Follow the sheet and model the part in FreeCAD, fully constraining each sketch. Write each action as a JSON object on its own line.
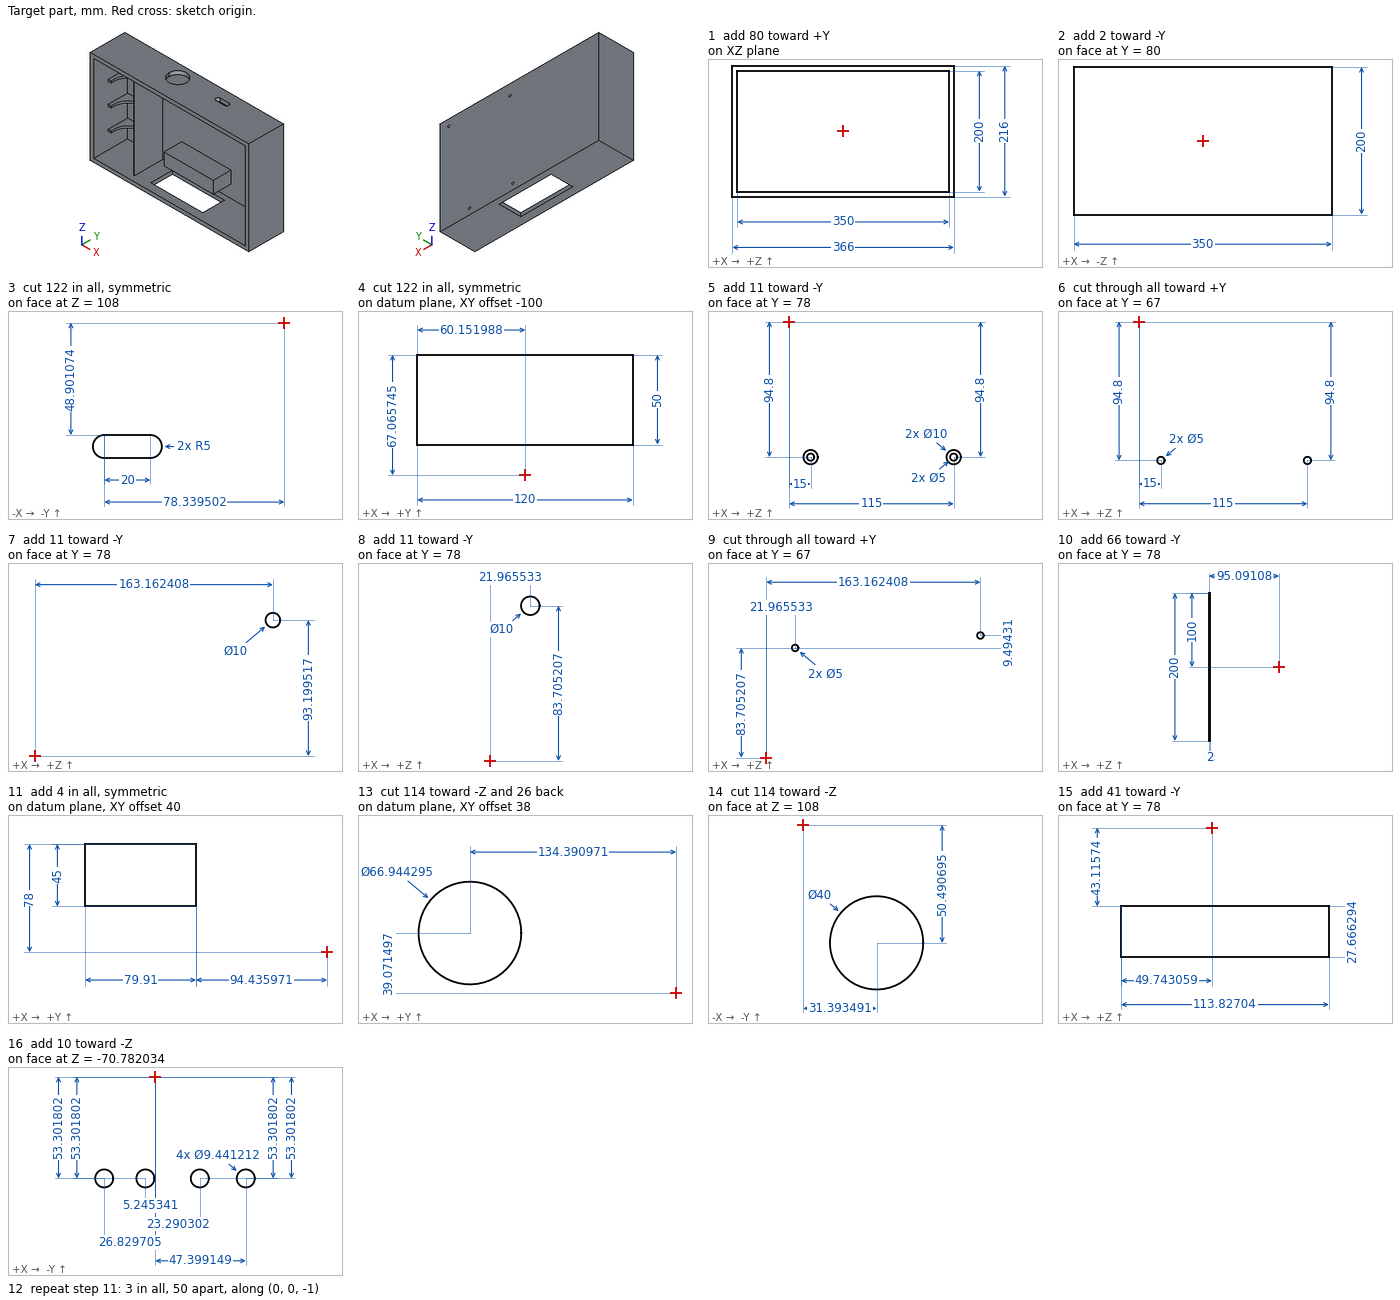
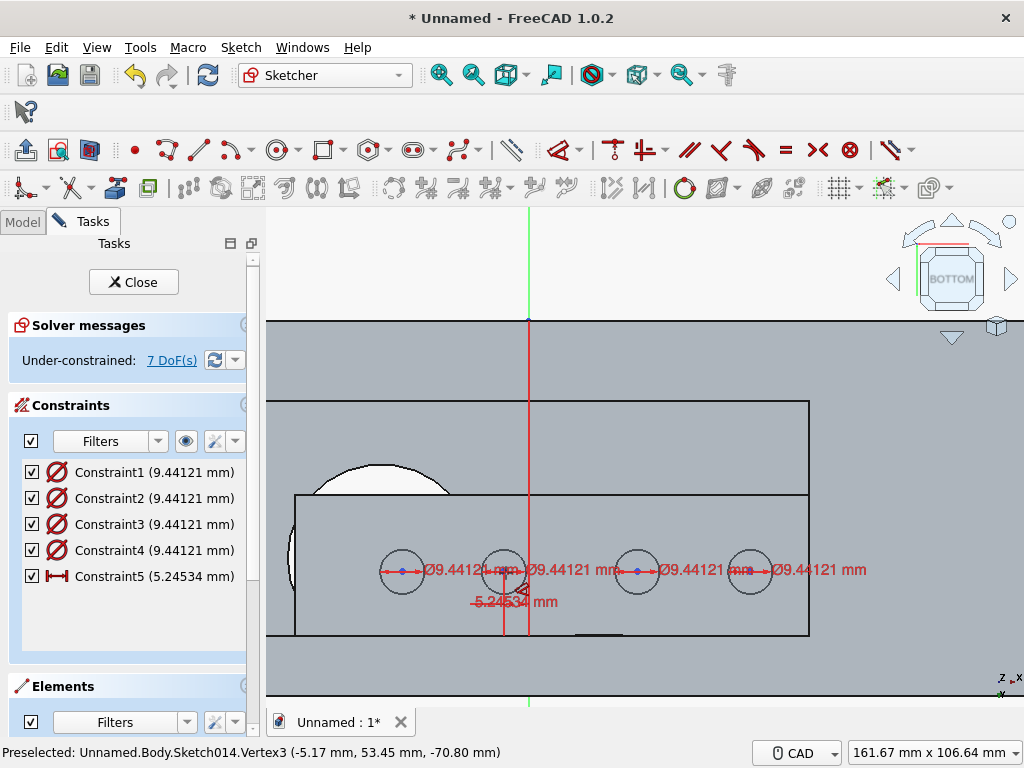
{"action": "left_click", "coordinate": [750, 572]}
{"action": "left_click", "coordinate": [639, 287]}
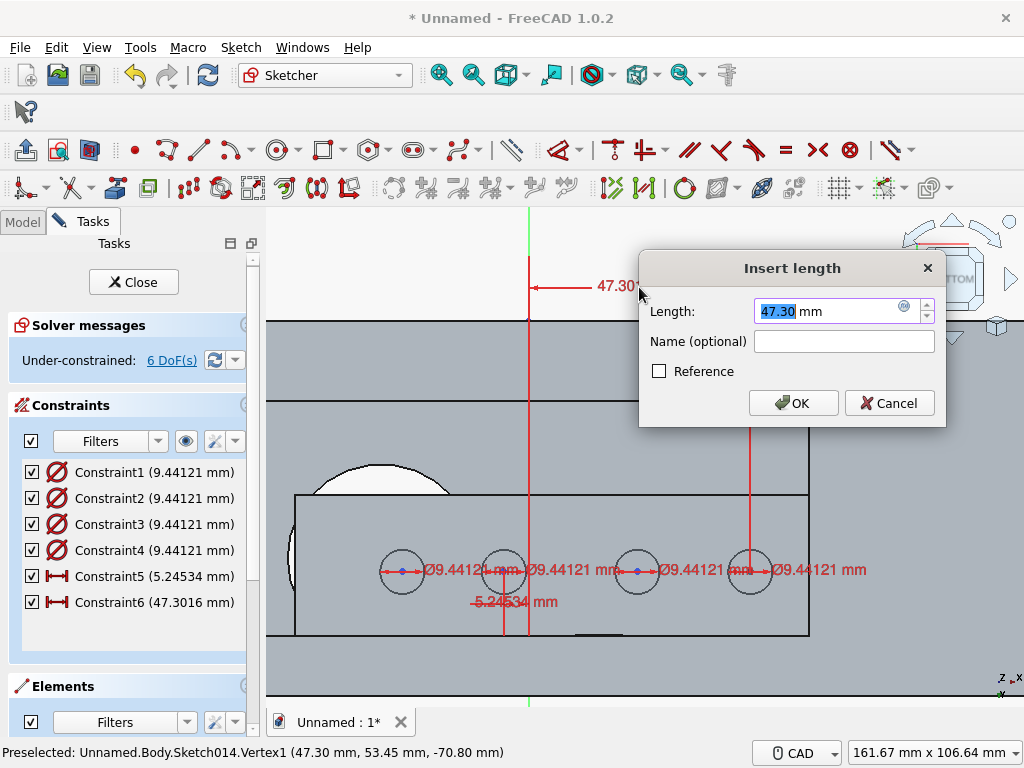
{"action": "type", "text": "47.399149"}
{"action": "key", "text": "Return"}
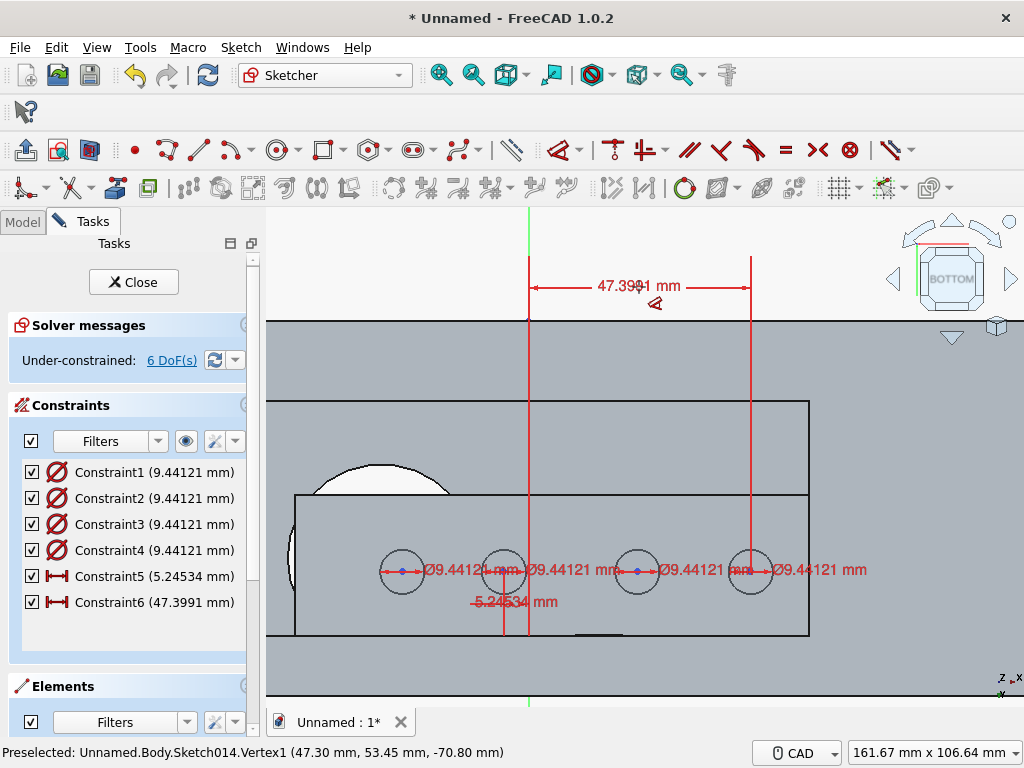
{"action": "left_click", "coordinate": [751, 572]}
{"action": "left_click", "coordinate": [785, 447]}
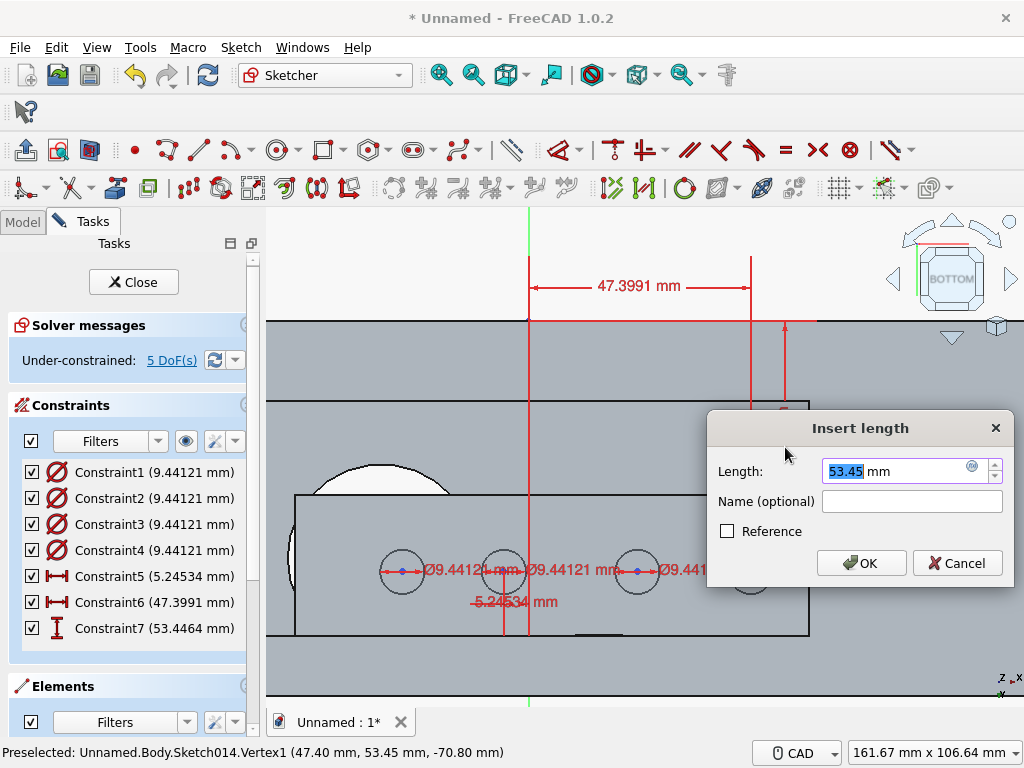
{"action": "type", "text": "53.301802"}
{"action": "key", "text": "Return"}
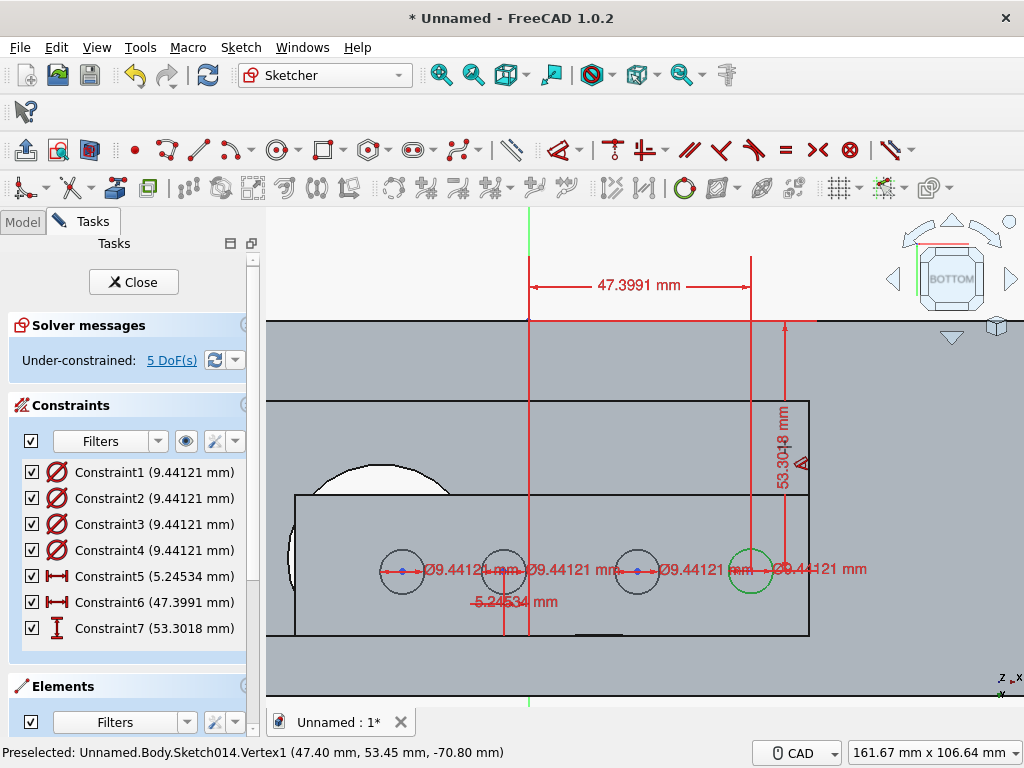
{"action": "left_click", "coordinate": [637, 572]}
{"action": "left_click", "coordinate": [558, 287]}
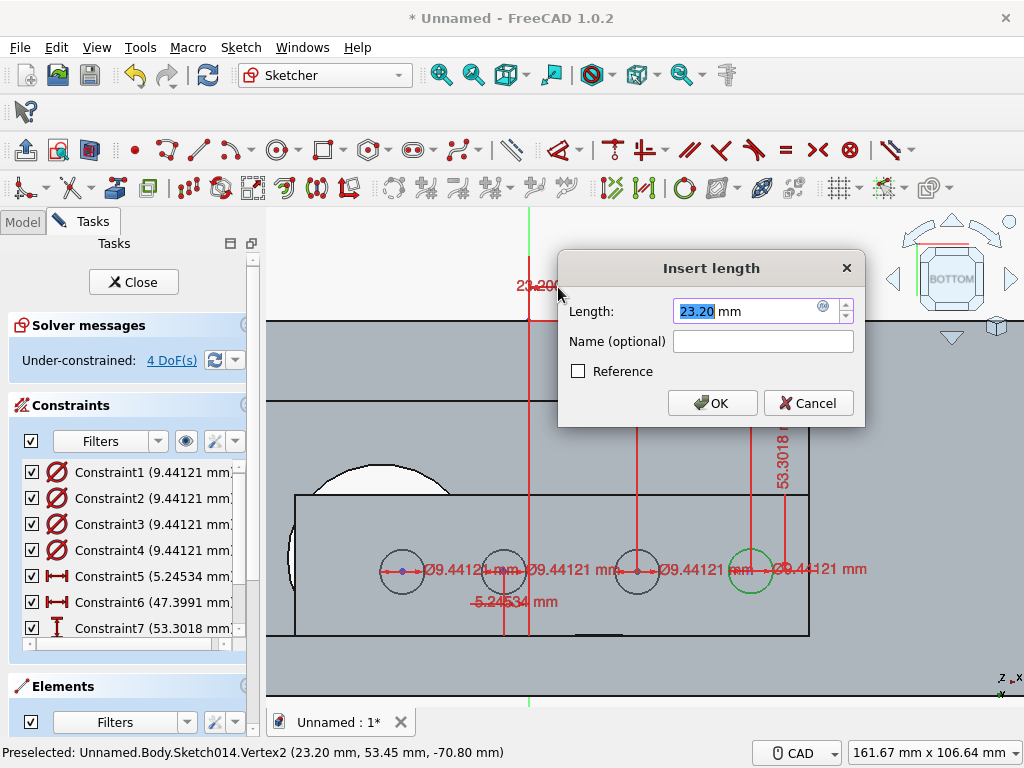
{"action": "type", "text": "23.290302"}
{"action": "key", "text": "Return"}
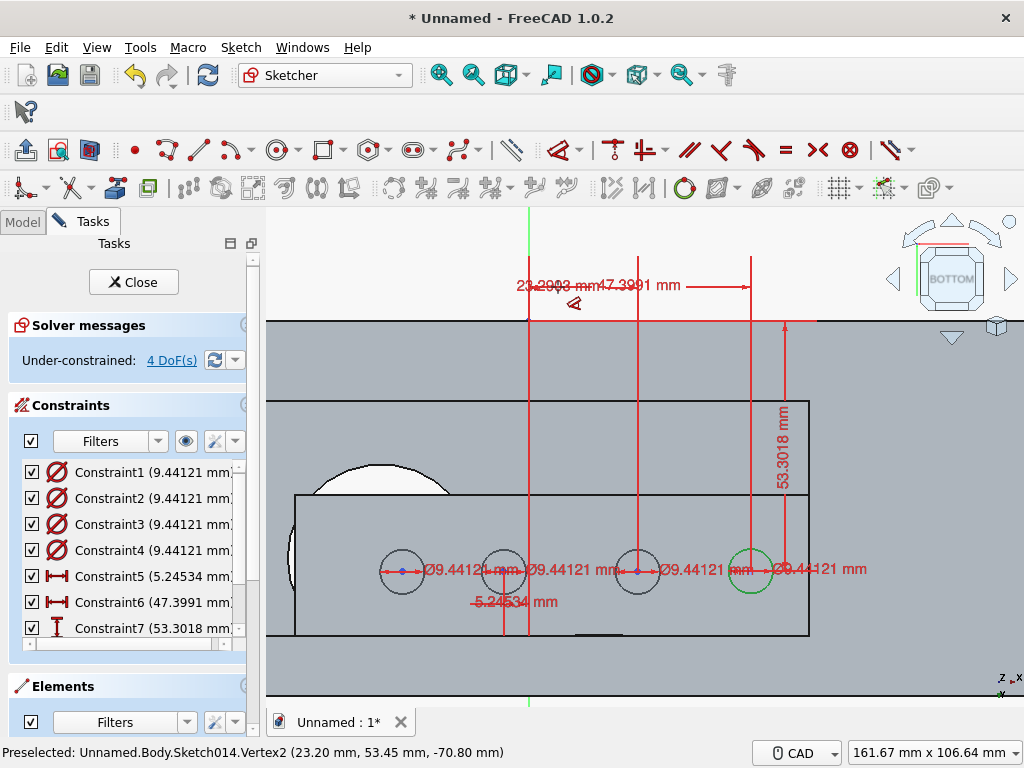
{"action": "left_click", "coordinate": [638, 572]}
{"action": "left_click", "coordinate": [672, 447]}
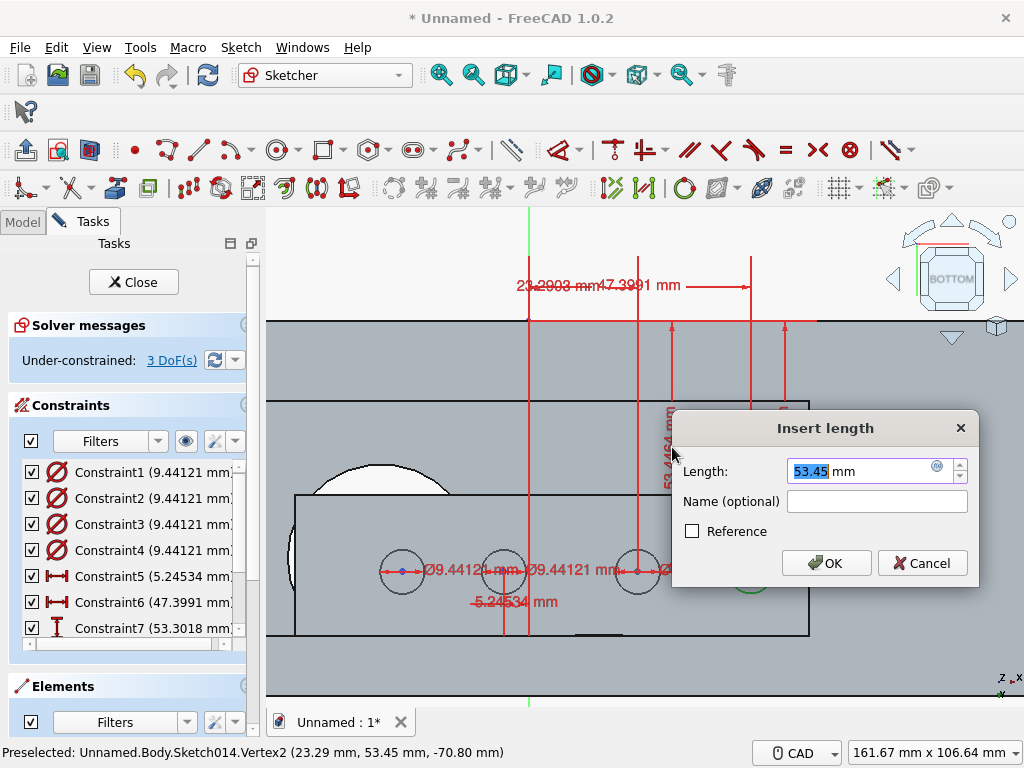
{"action": "type", "text": "53.301802"}
{"action": "key", "text": "Return"}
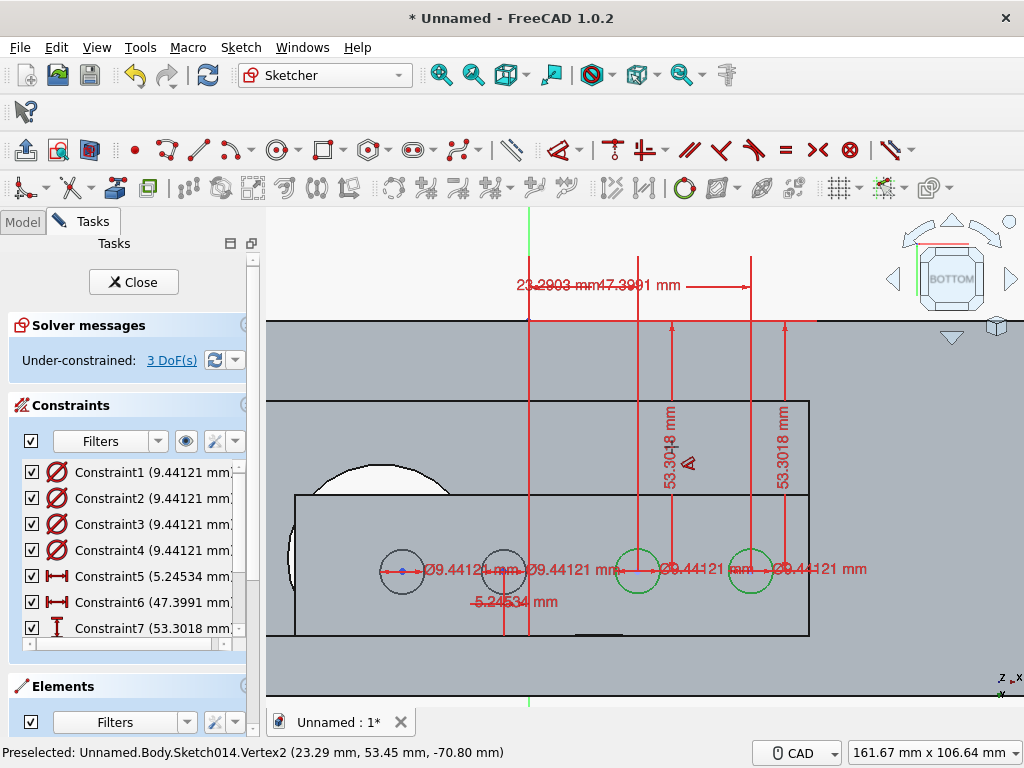
{"action": "left_click", "coordinate": [504, 572]}
{"action": "left_click", "coordinate": [470, 447]}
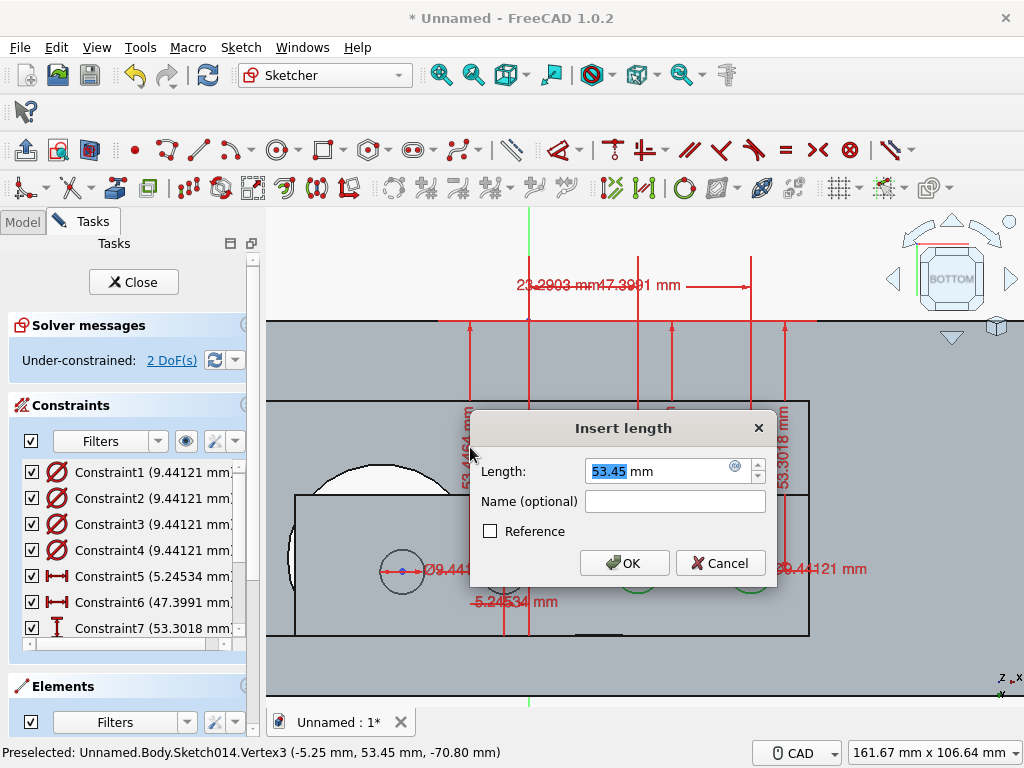
{"action": "type", "text": "53.301802"}
{"action": "key", "text": "Return"}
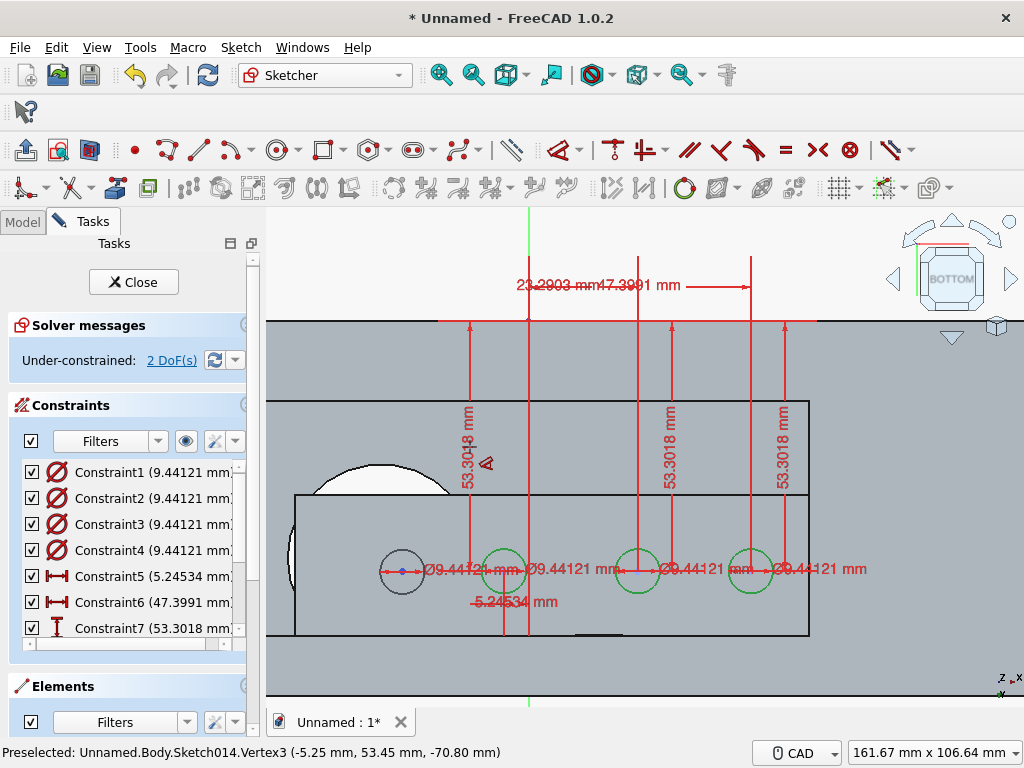
{"action": "left_click", "coordinate": [402, 572]}
{"action": "left_click", "coordinate": [465, 287]}